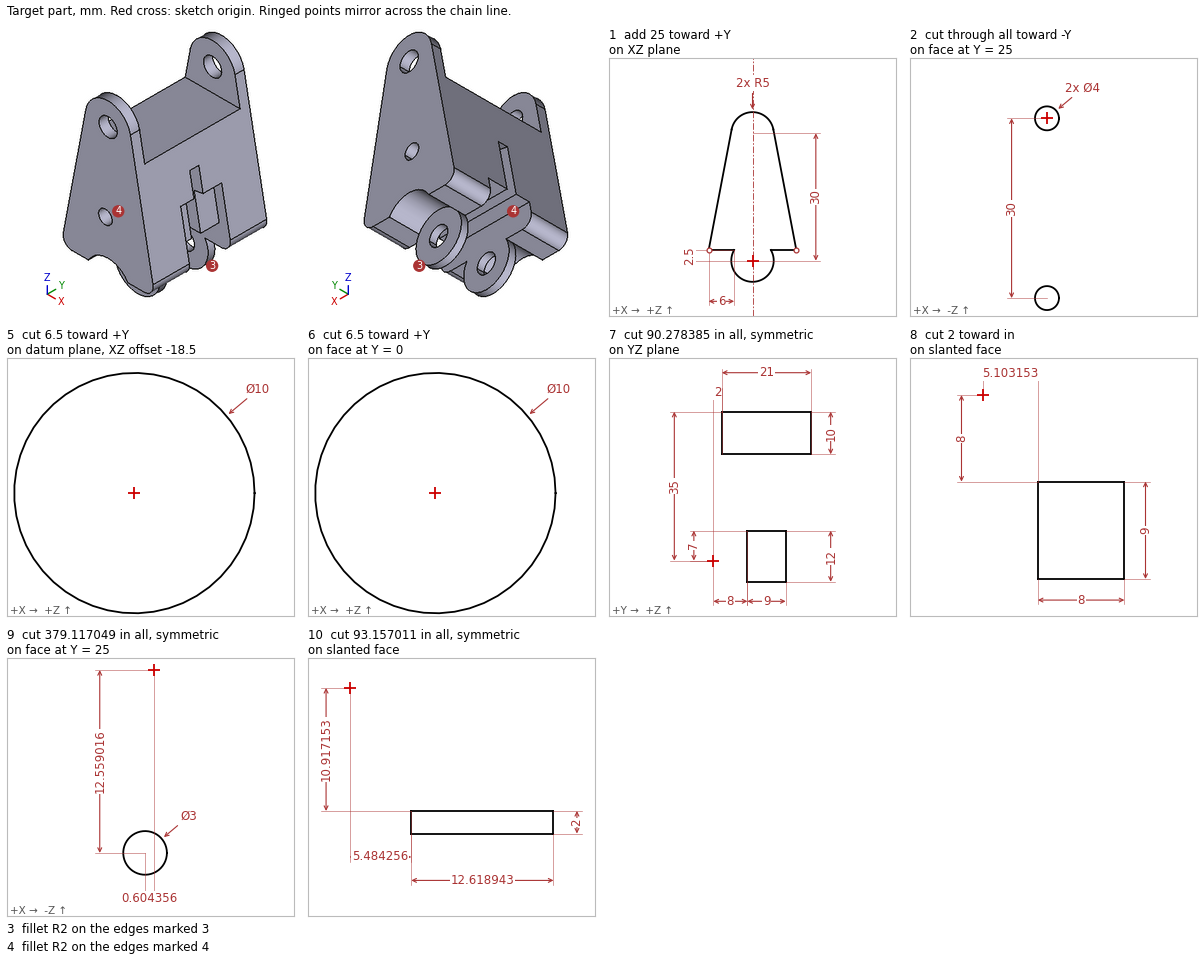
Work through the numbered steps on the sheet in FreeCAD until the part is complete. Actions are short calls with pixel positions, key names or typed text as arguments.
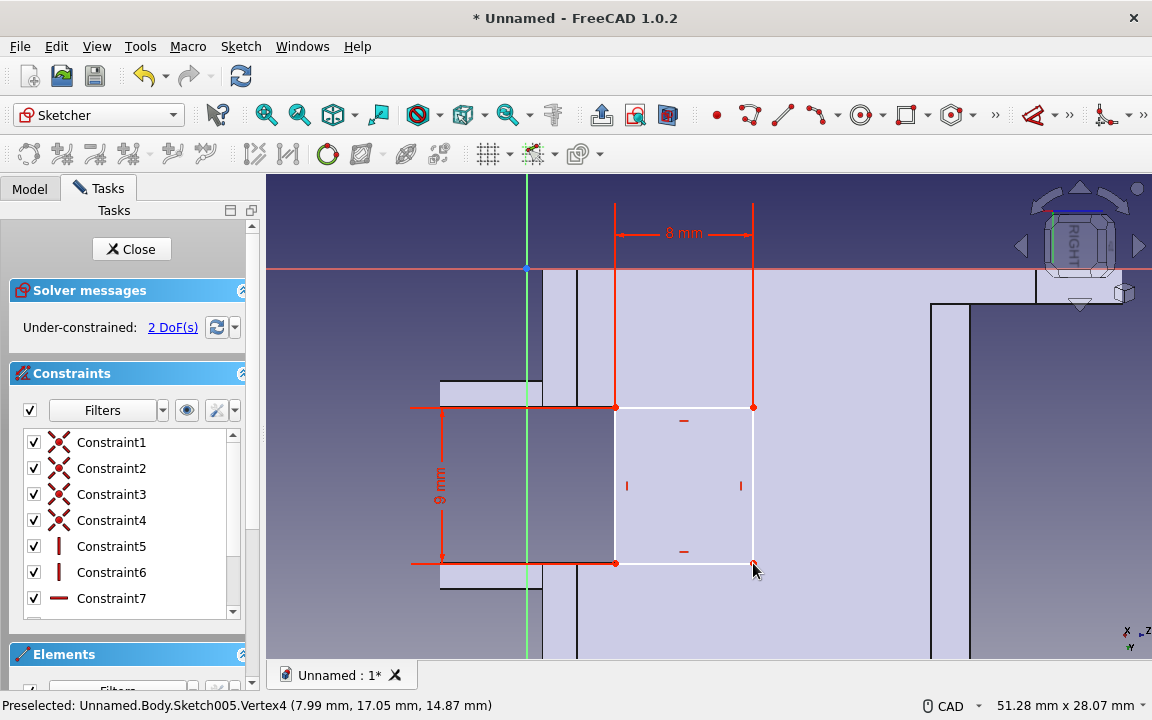
key(d)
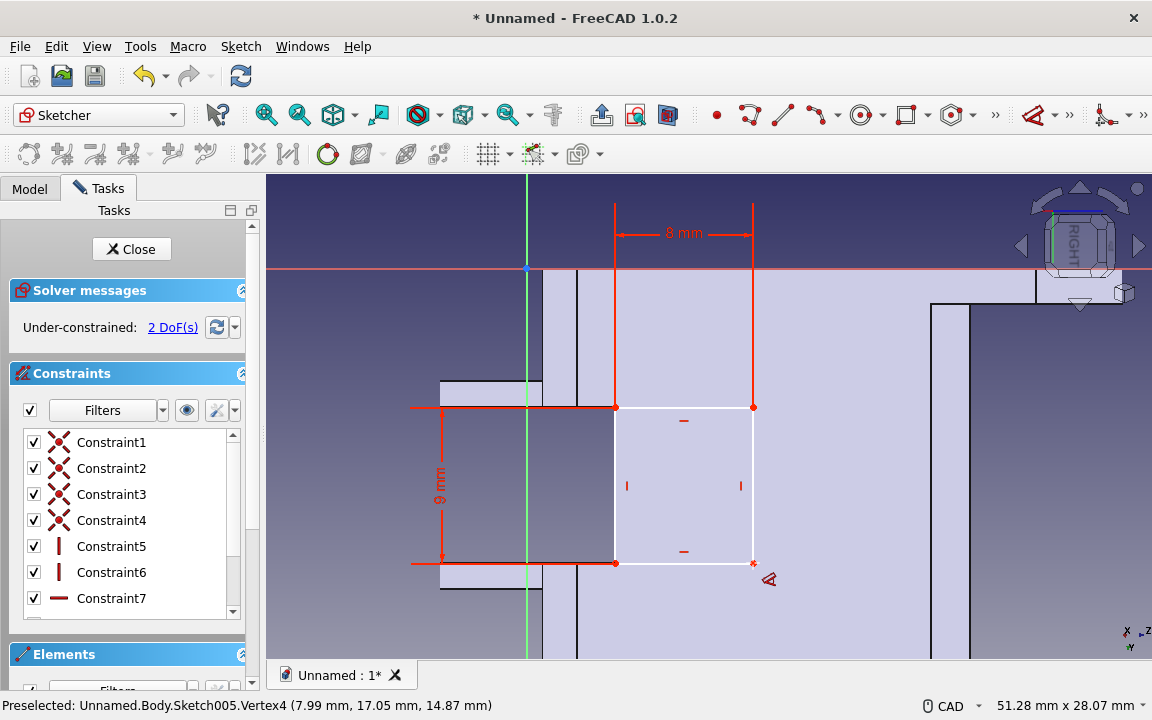
click(615, 408)
click(493, 338)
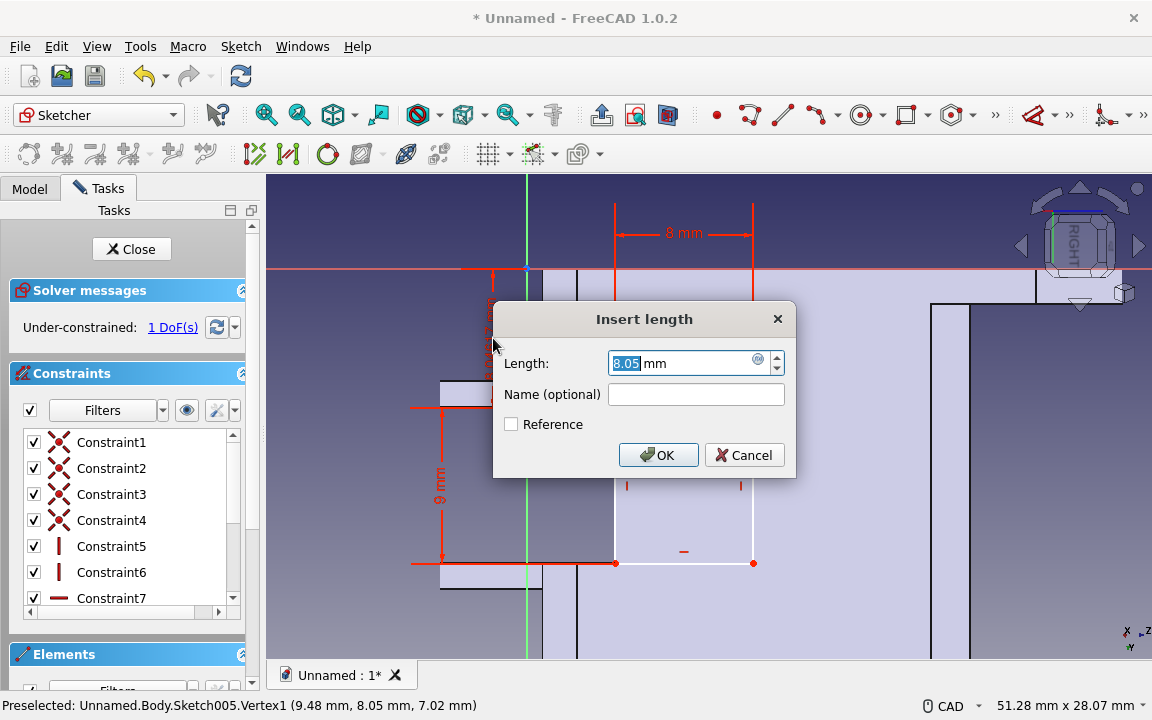
text(8)
key(Return)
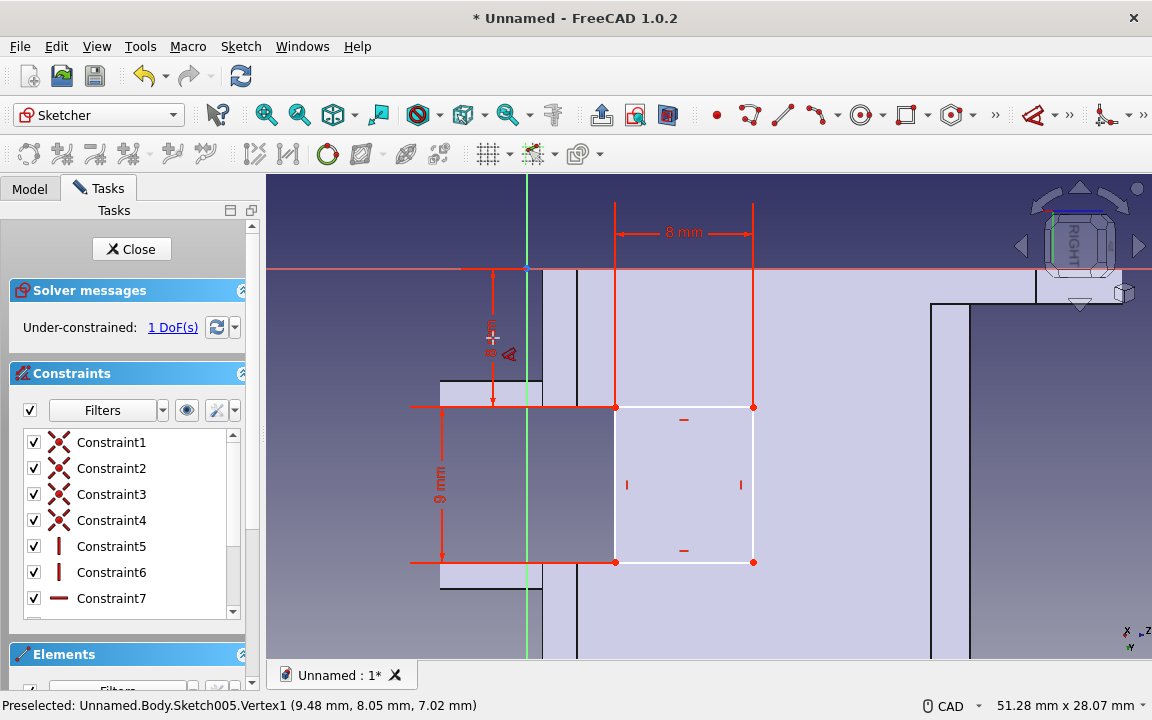
click(615, 407)
click(571, 235)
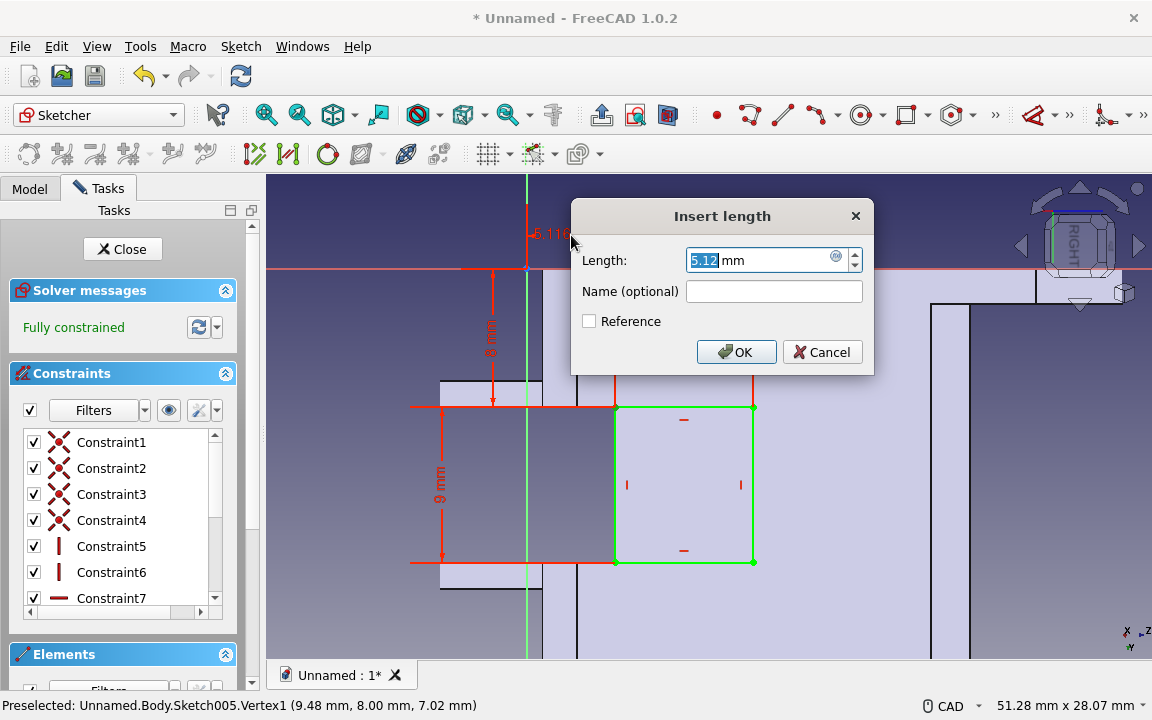
text(5.103153)
key(Return)
key(Escape)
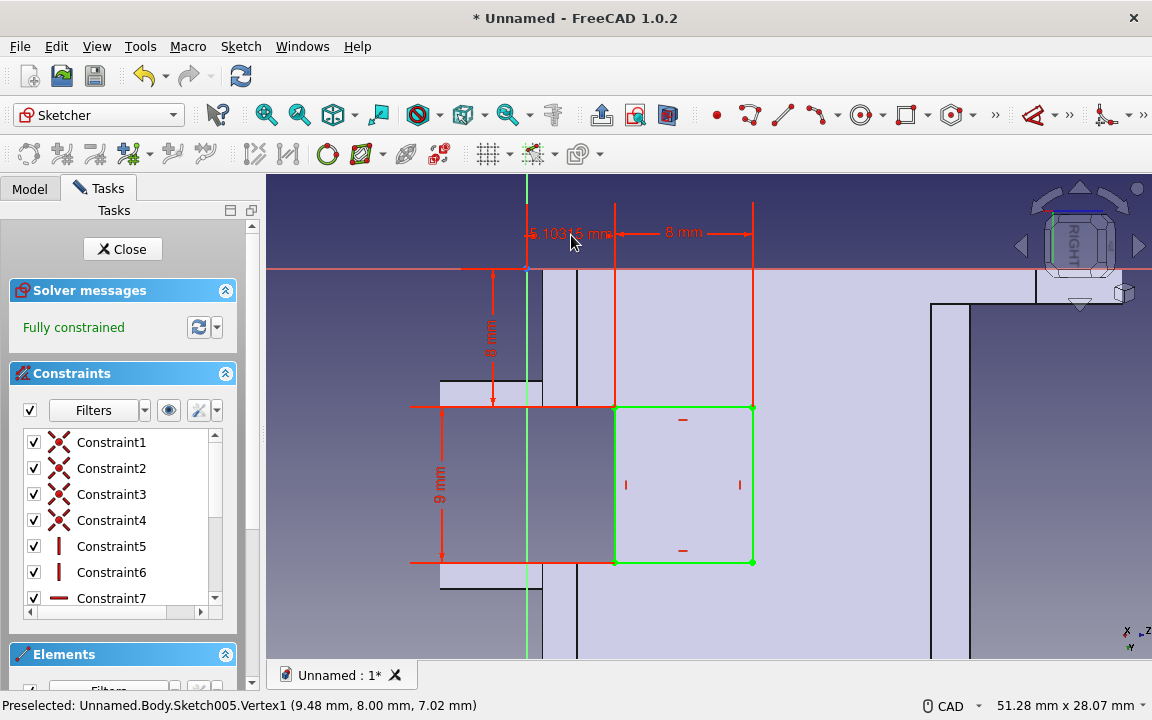
click(123, 249)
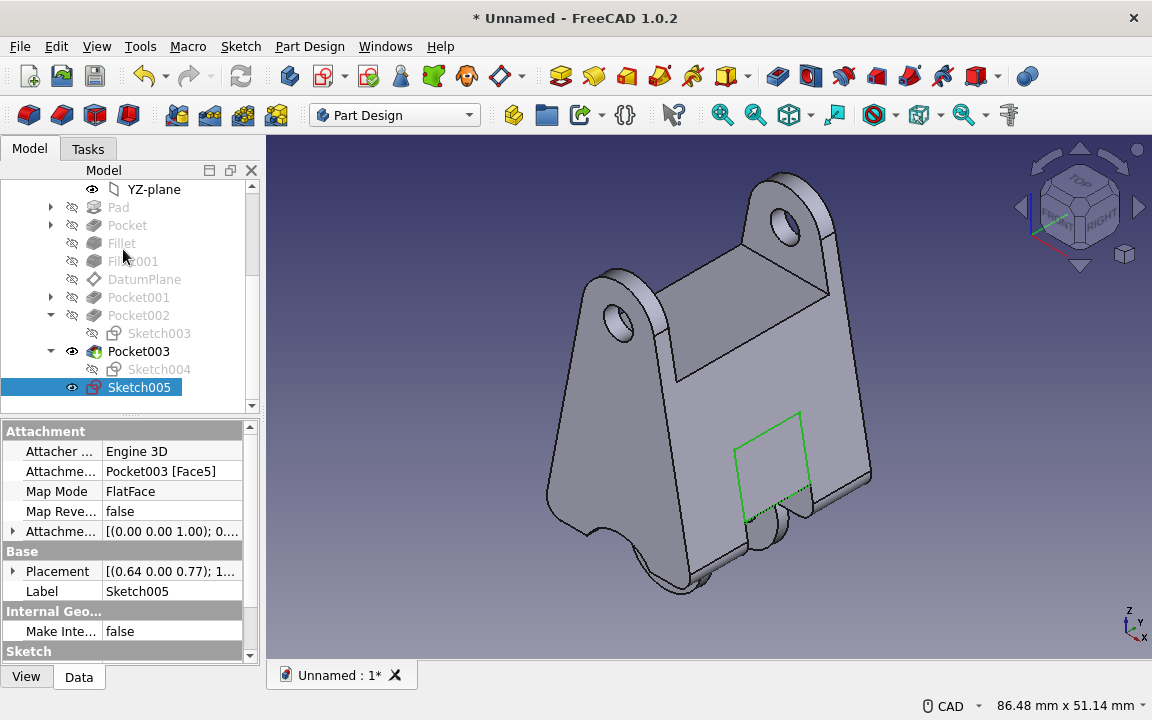
click(778, 76)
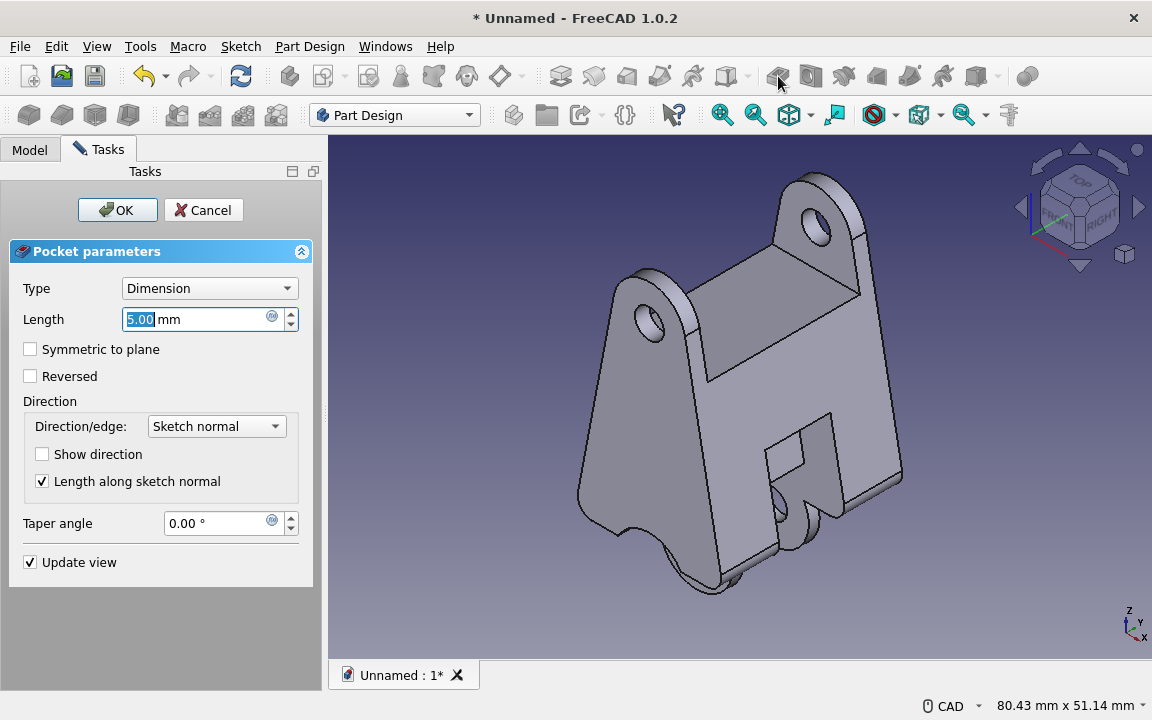
text(2)
key(Tab)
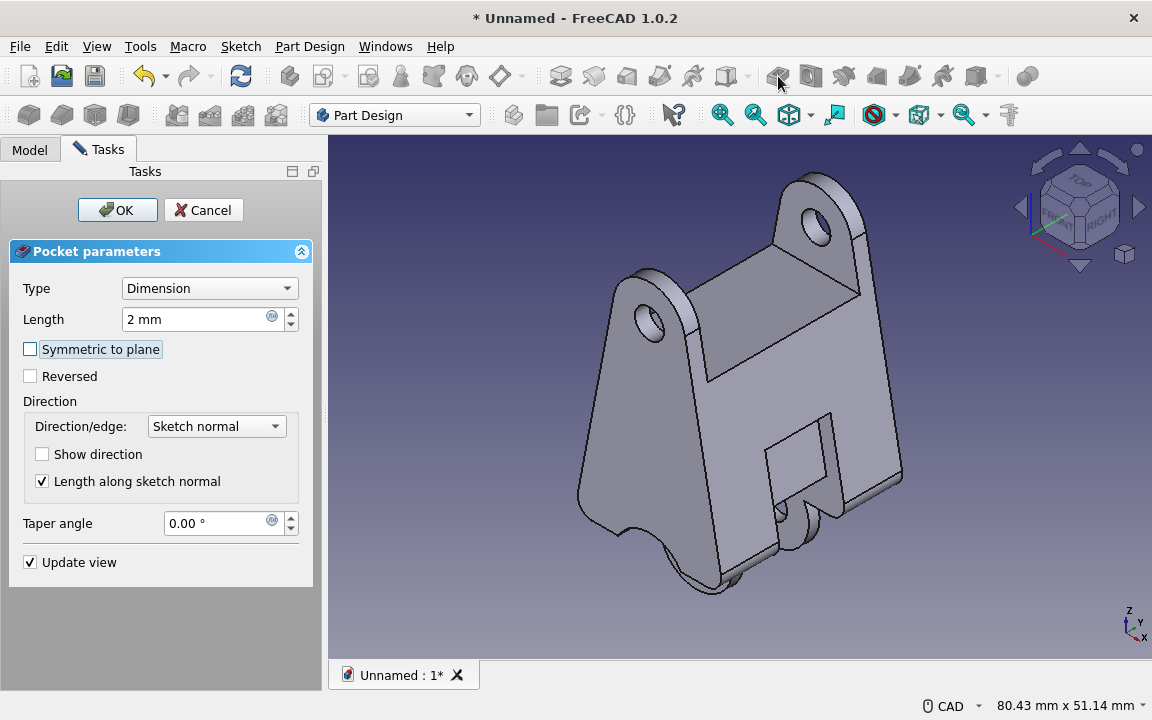
click(118, 210)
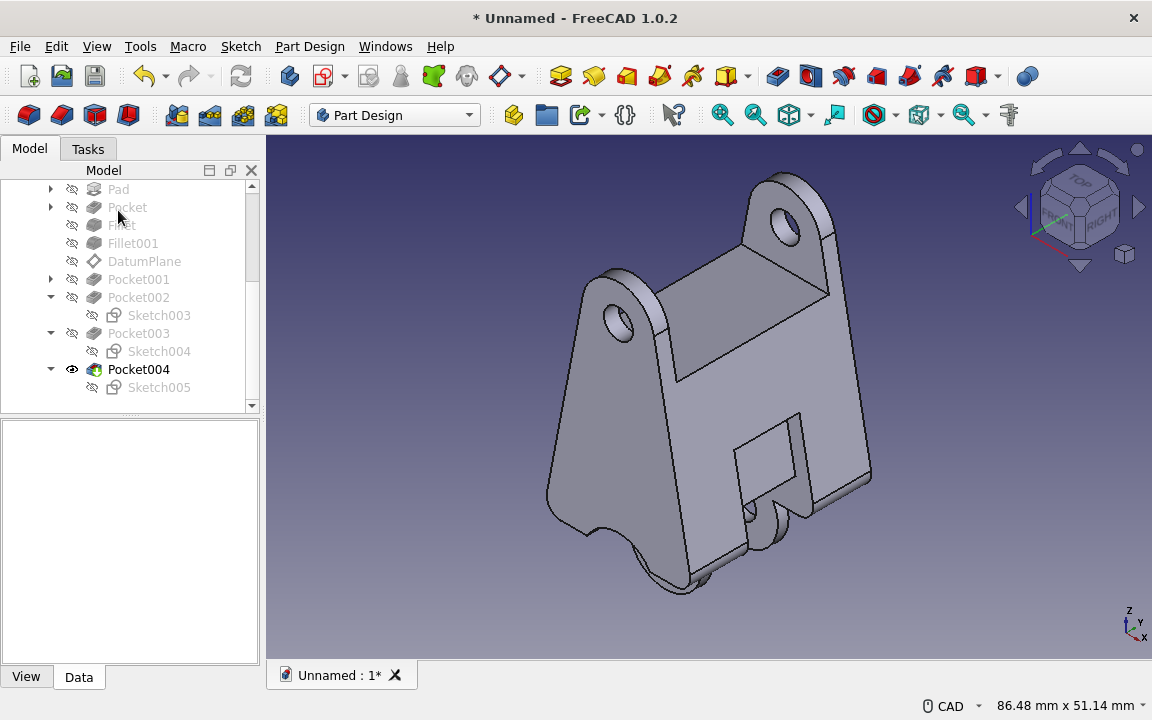
key(4)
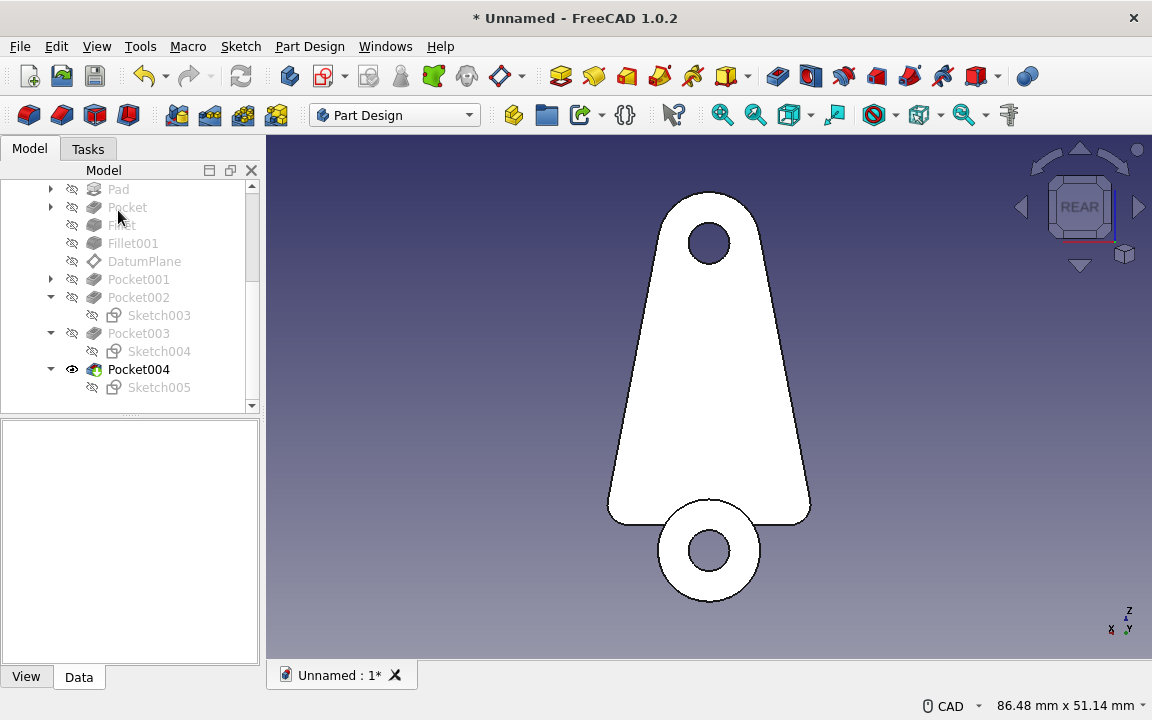
click(709, 405)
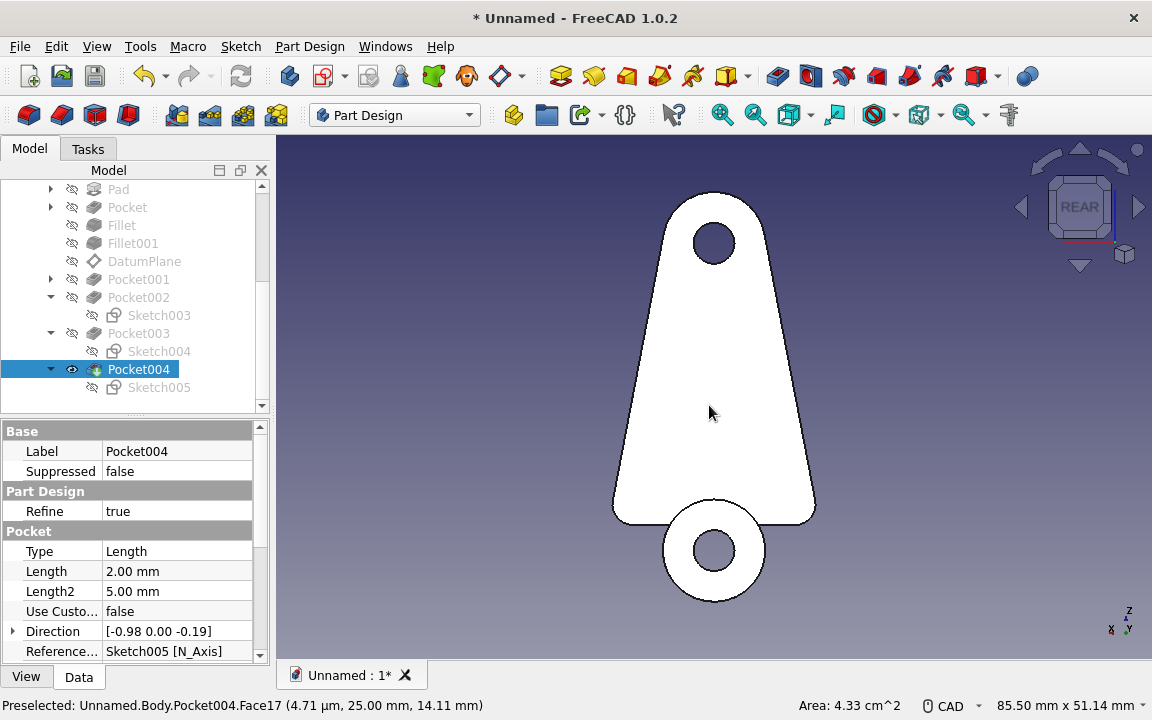
click(322, 76)